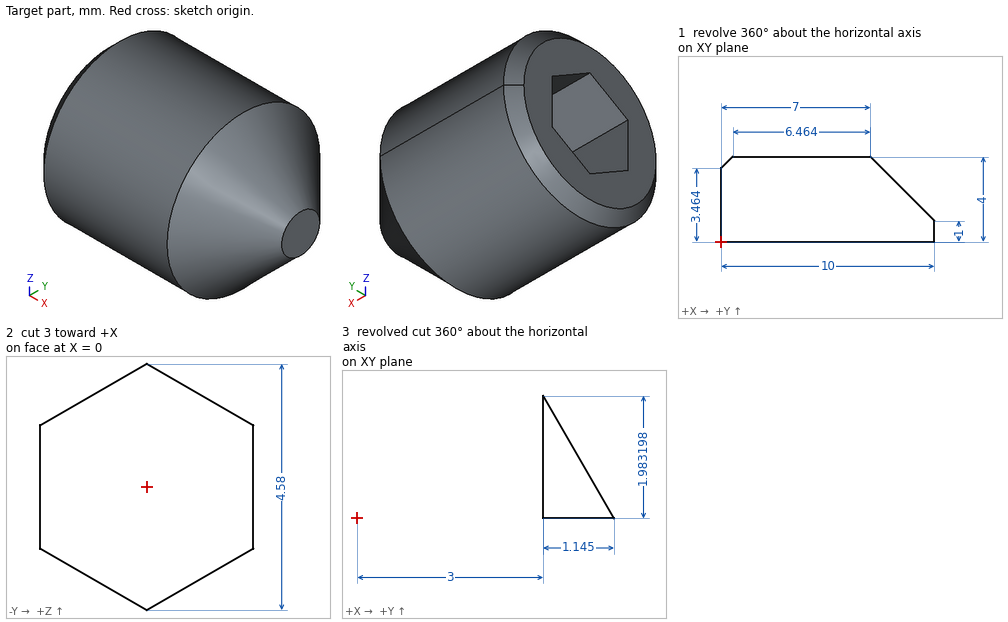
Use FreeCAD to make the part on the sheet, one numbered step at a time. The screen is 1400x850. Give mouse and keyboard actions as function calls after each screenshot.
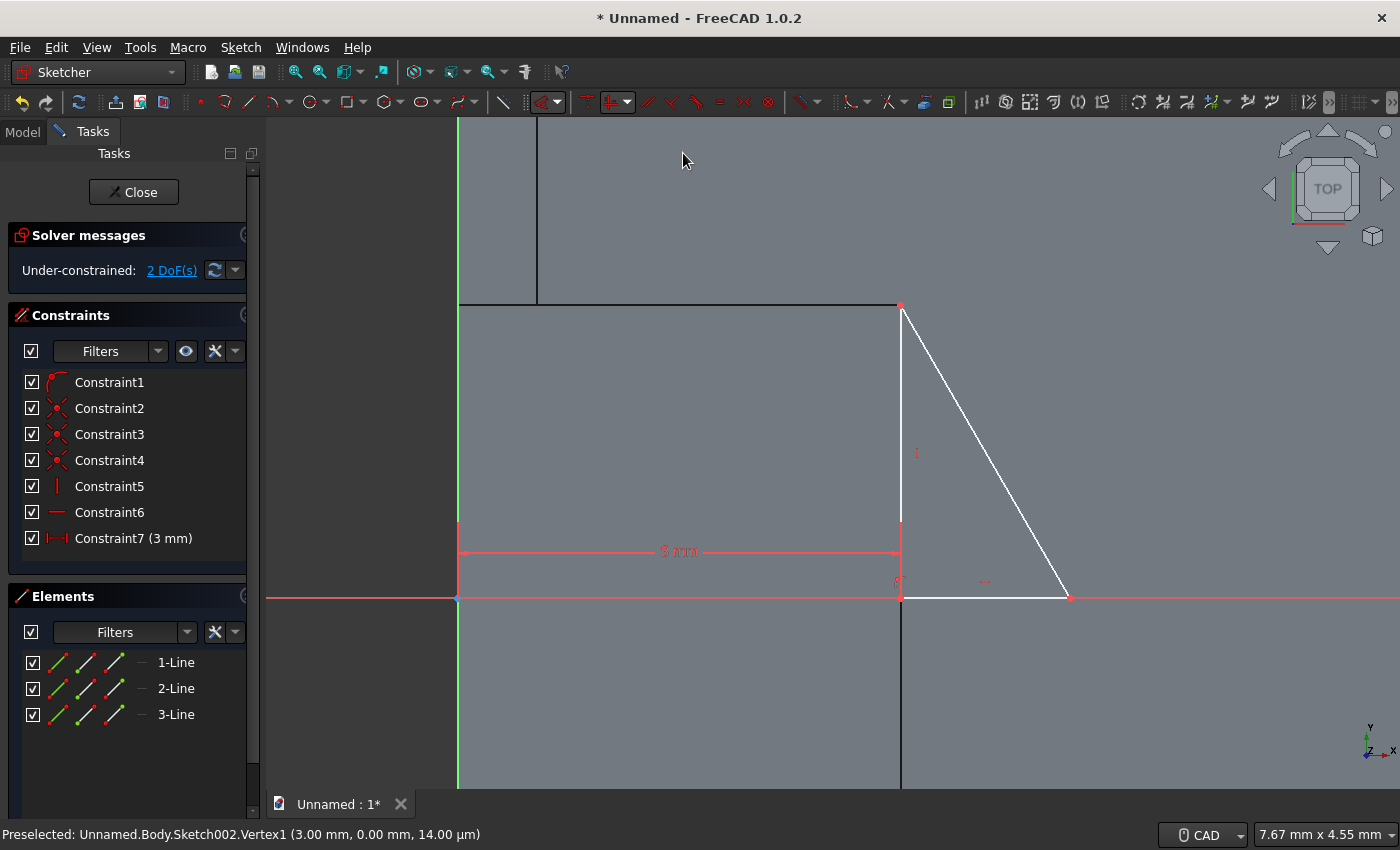
click(952, 598)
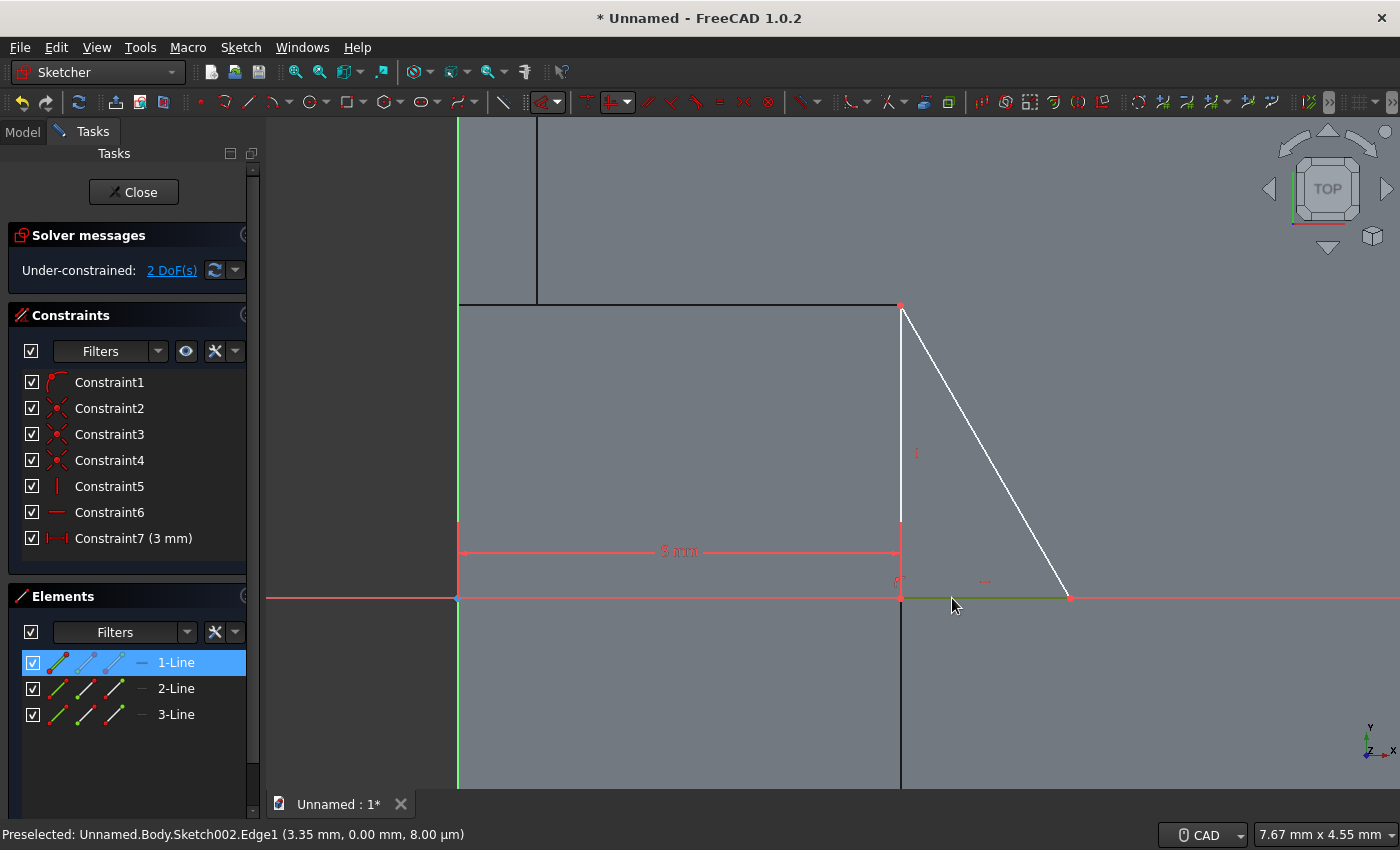
click(560, 102)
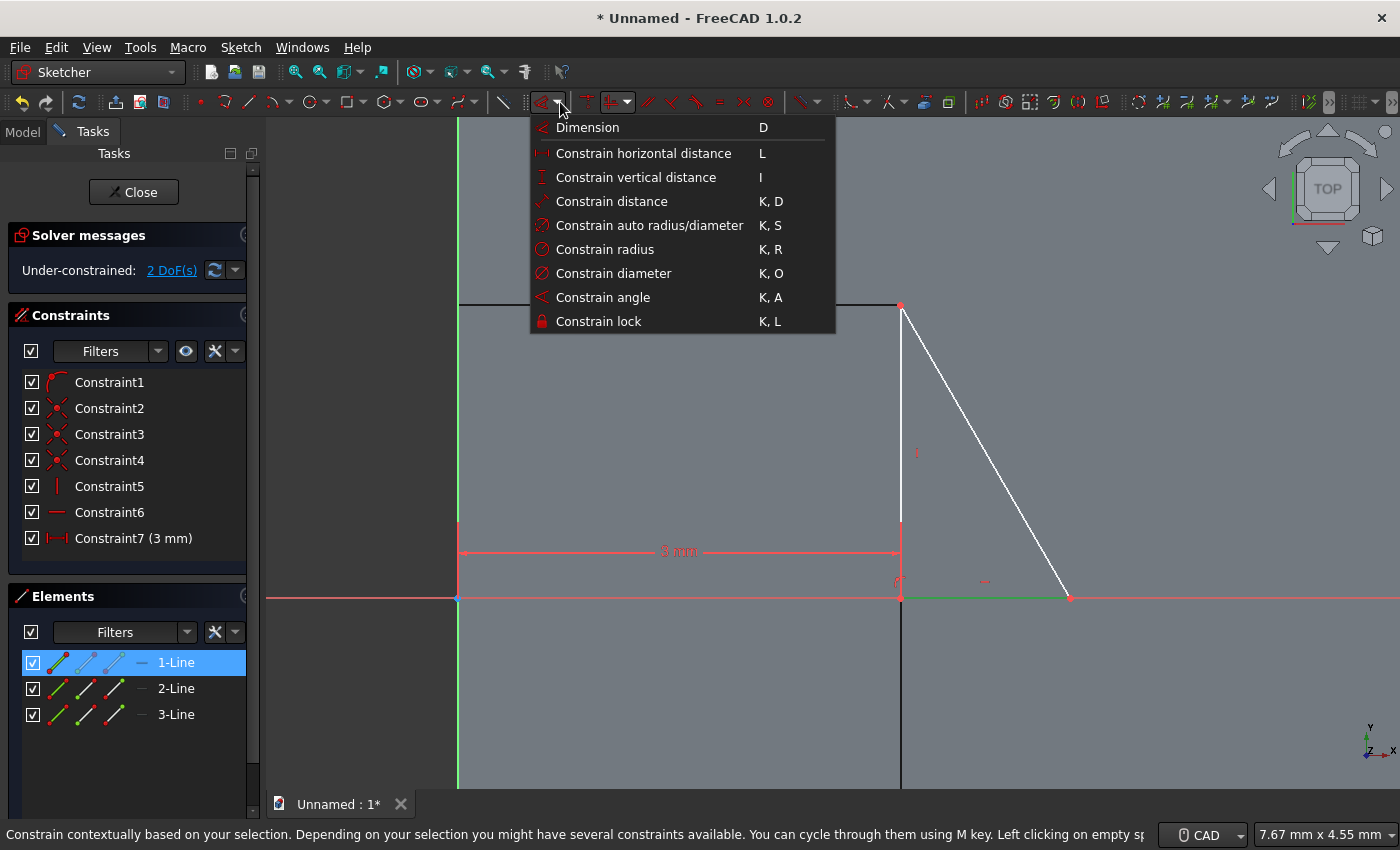
click(683, 153)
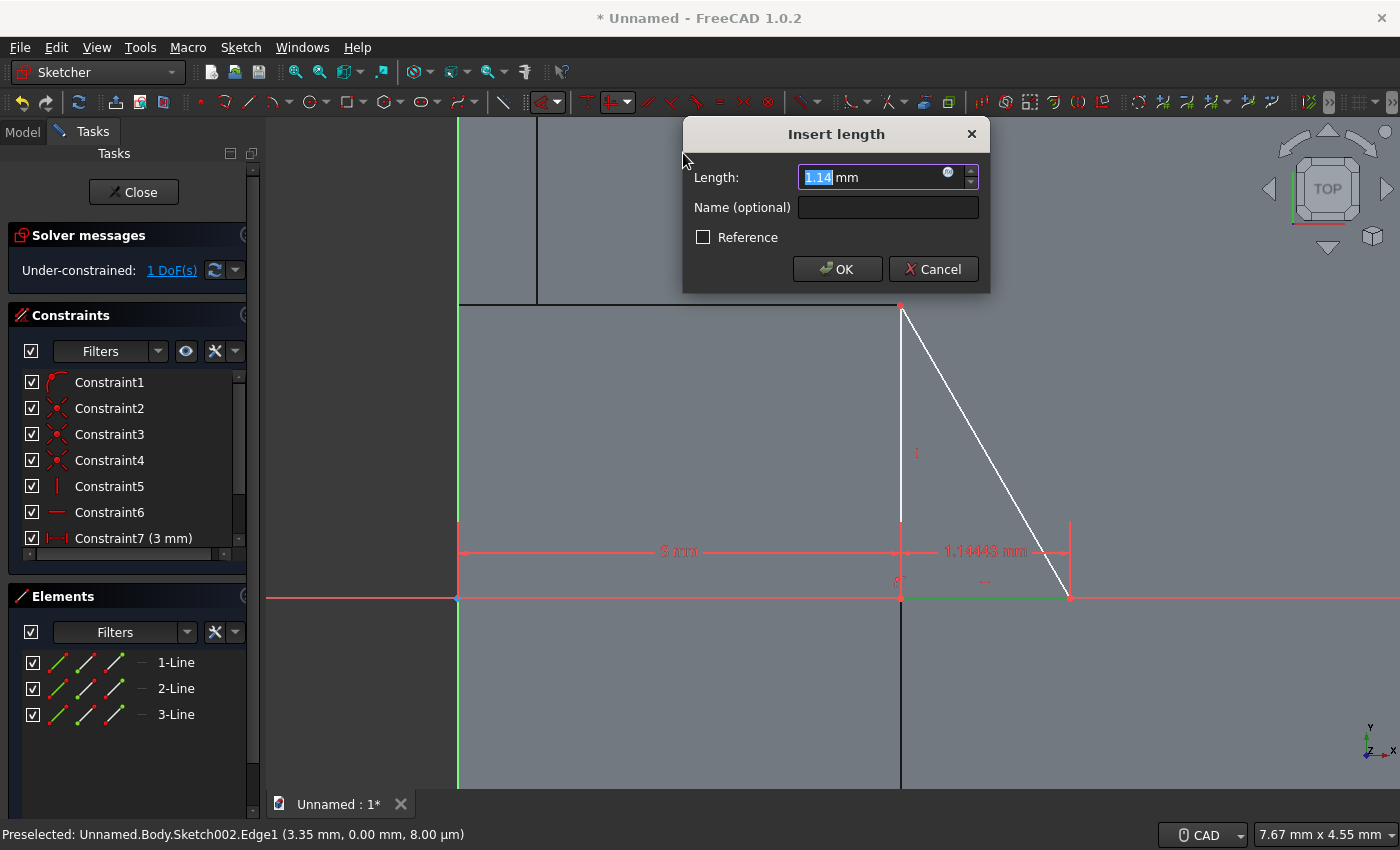
text(1.145)
key(Return)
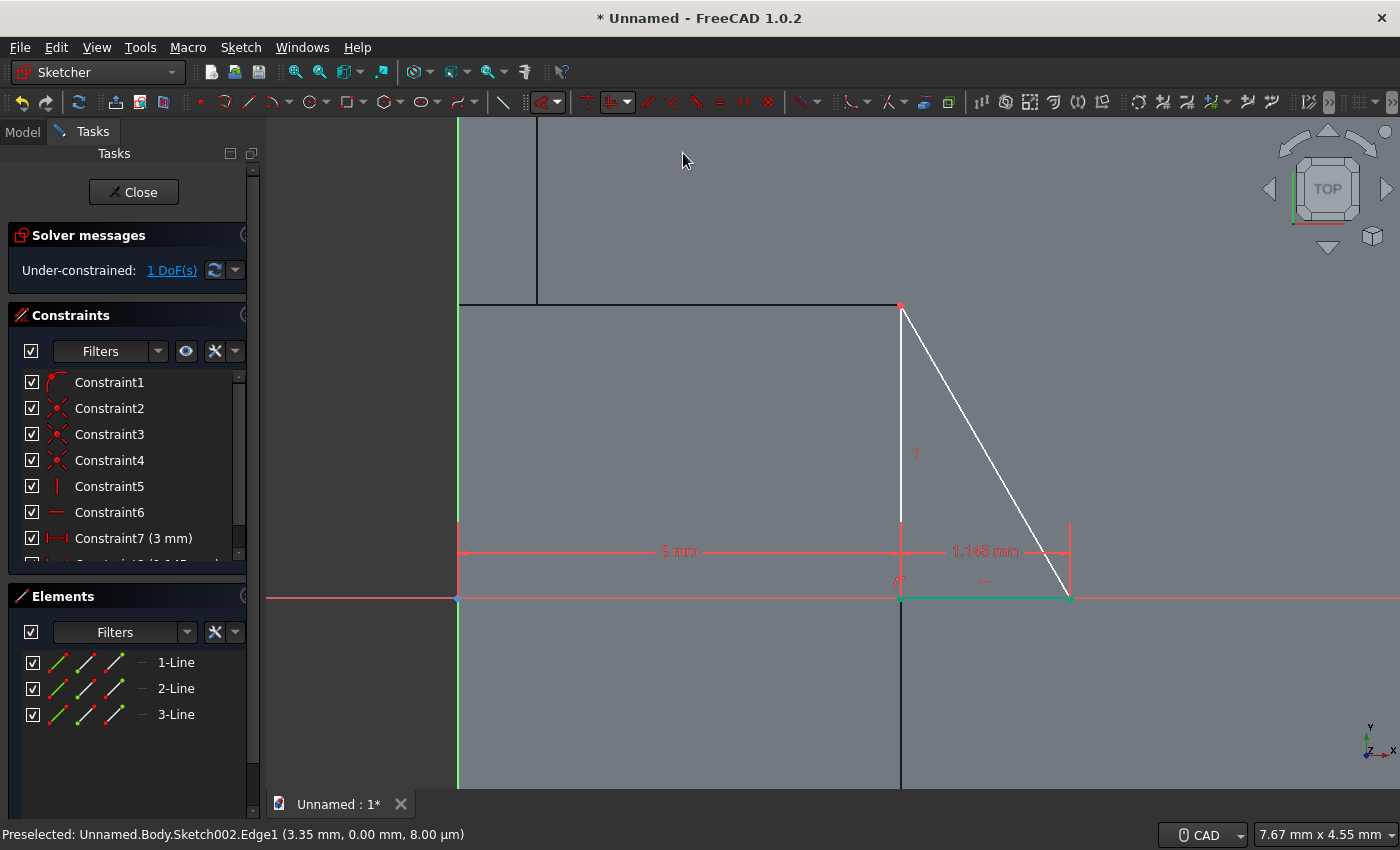
click(901, 394)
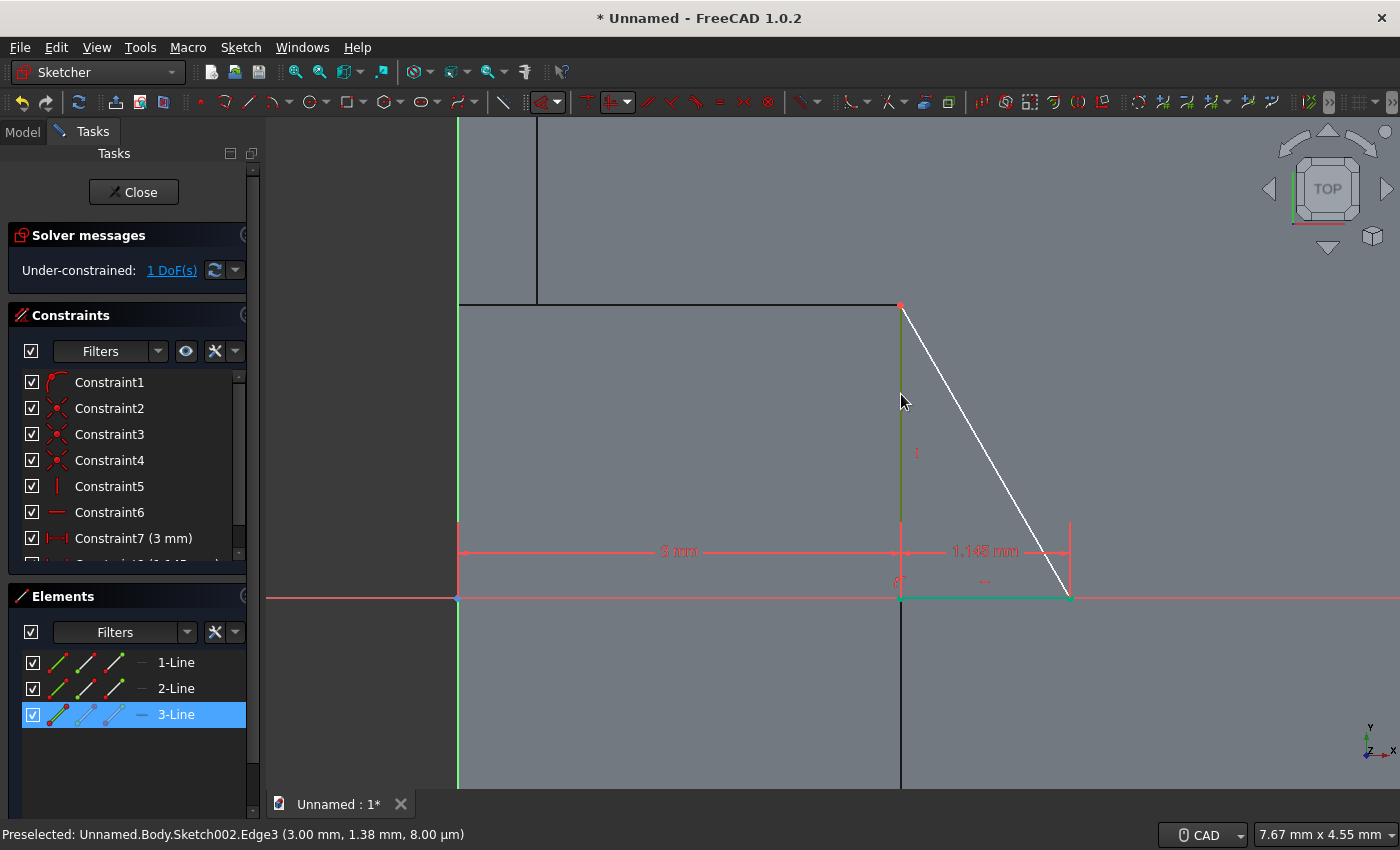
key(i)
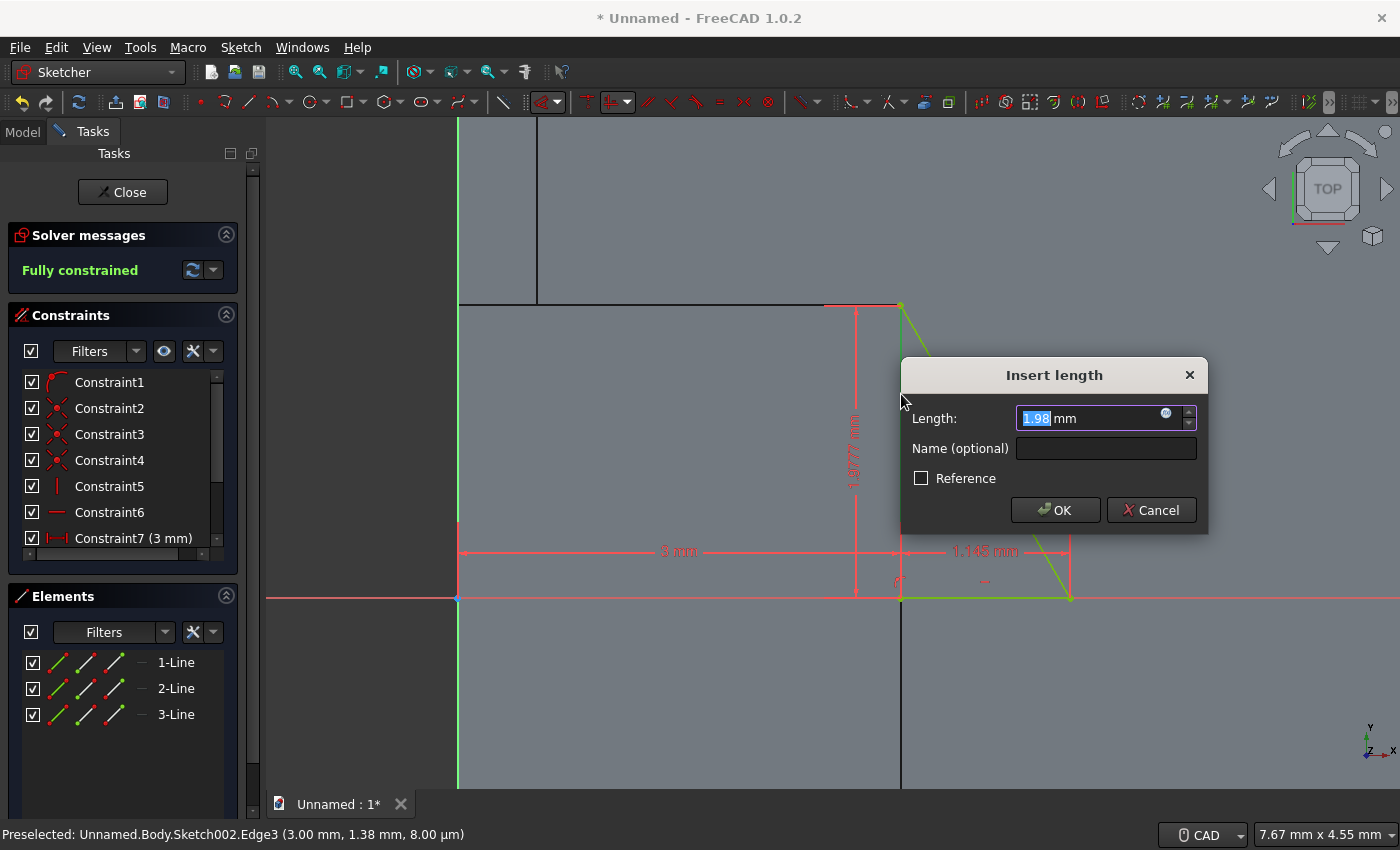
text(1.983198)
key(Return)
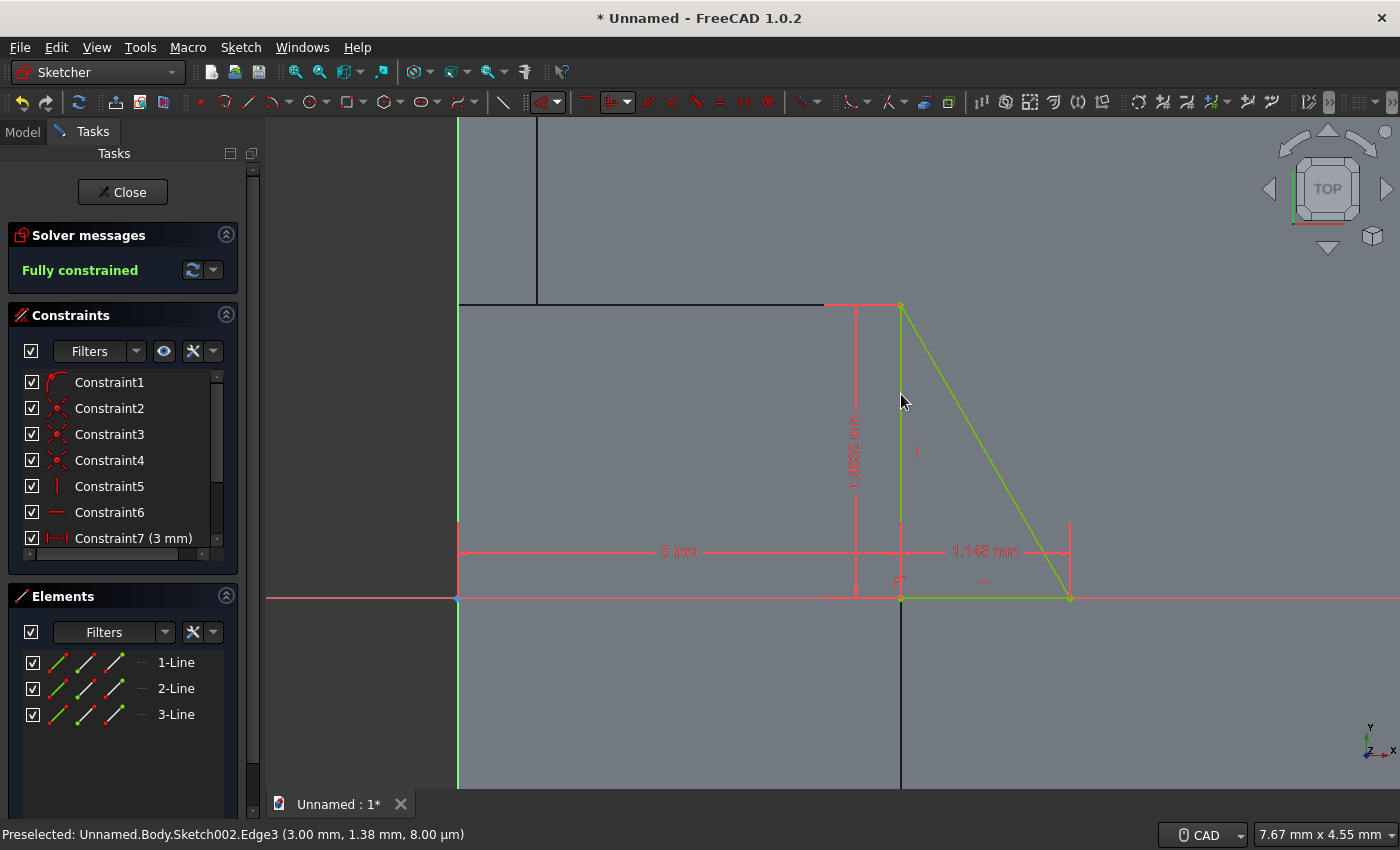
click(123, 192)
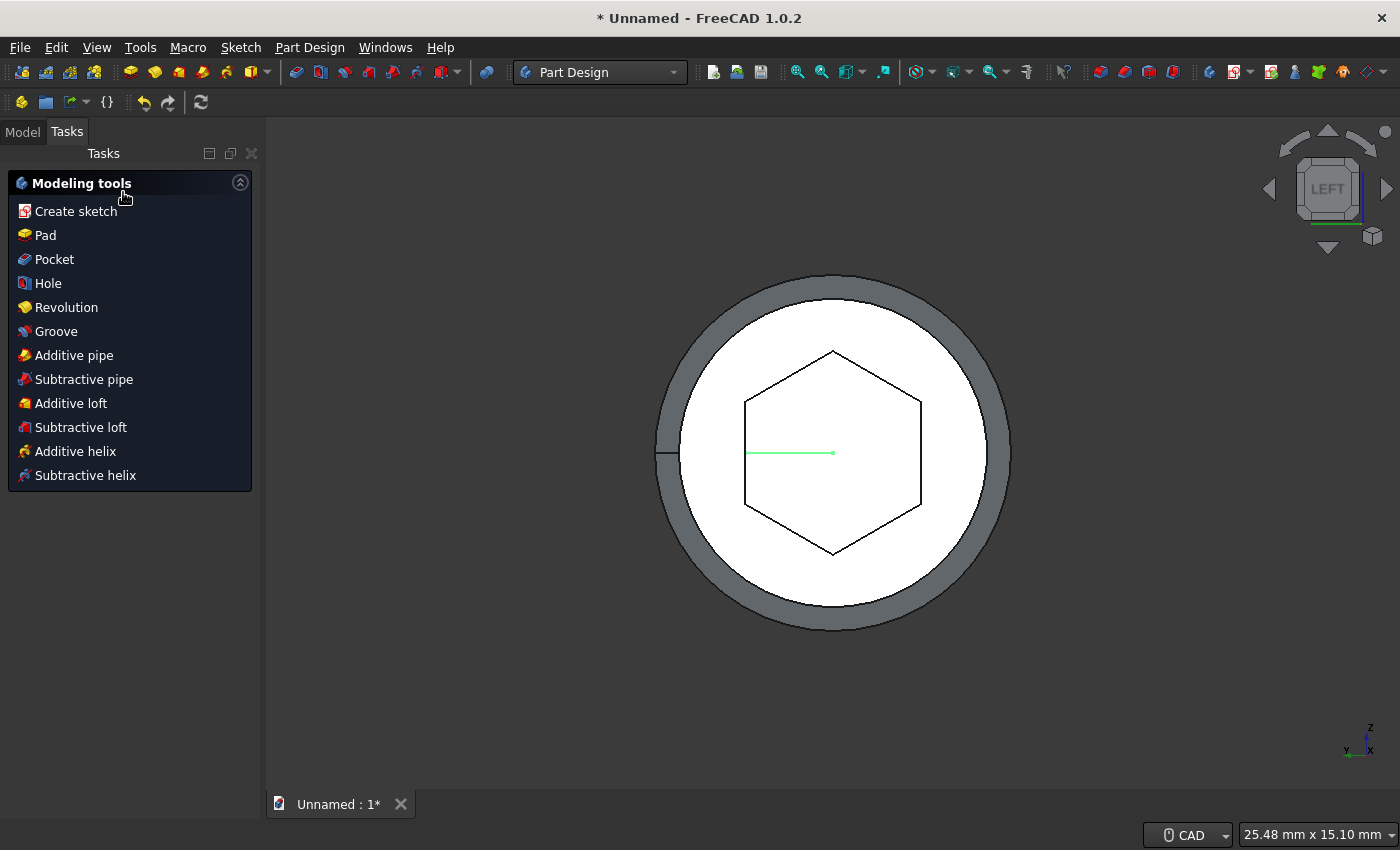
click(346, 72)